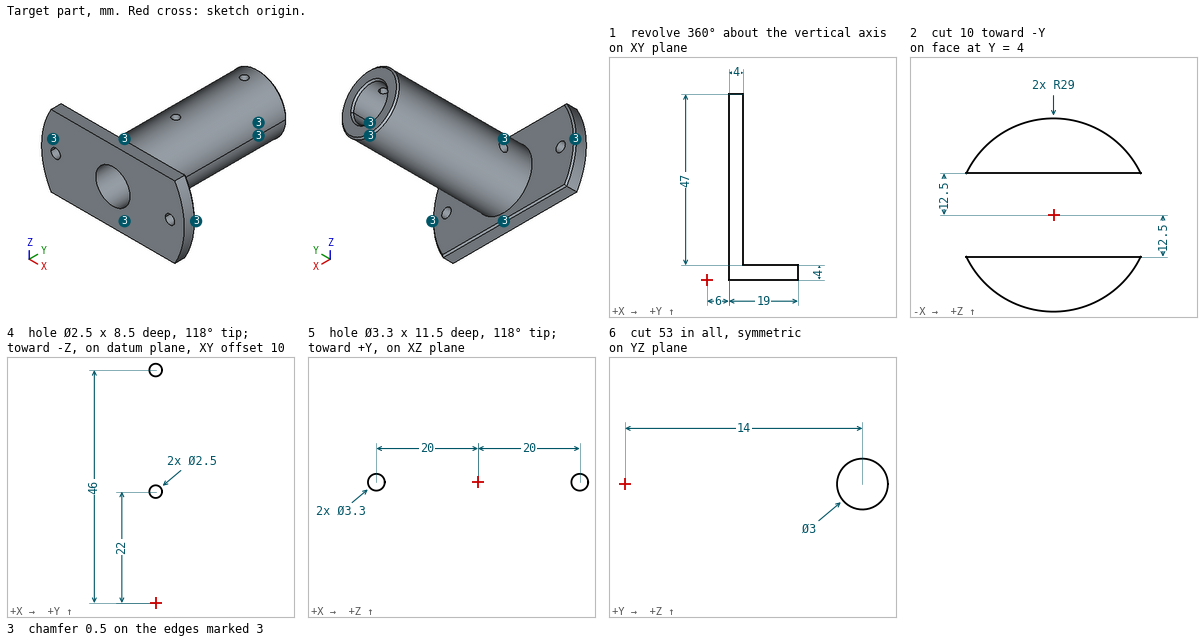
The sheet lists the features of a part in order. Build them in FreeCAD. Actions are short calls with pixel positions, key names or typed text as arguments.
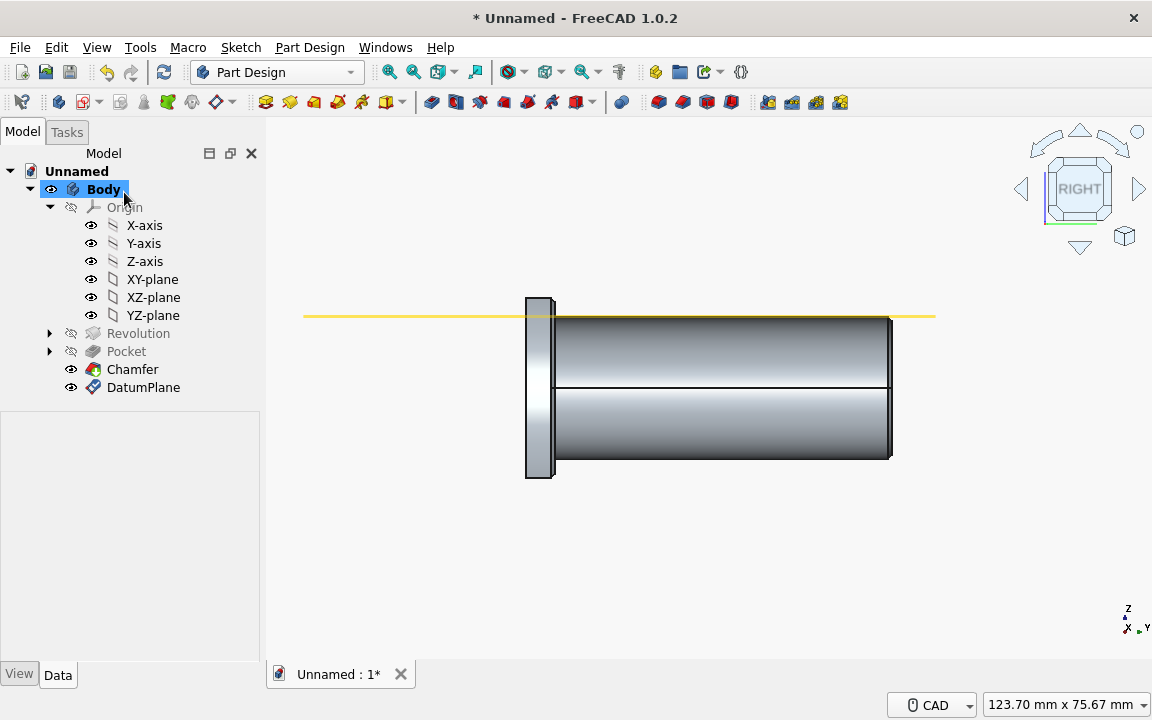
click(116, 387)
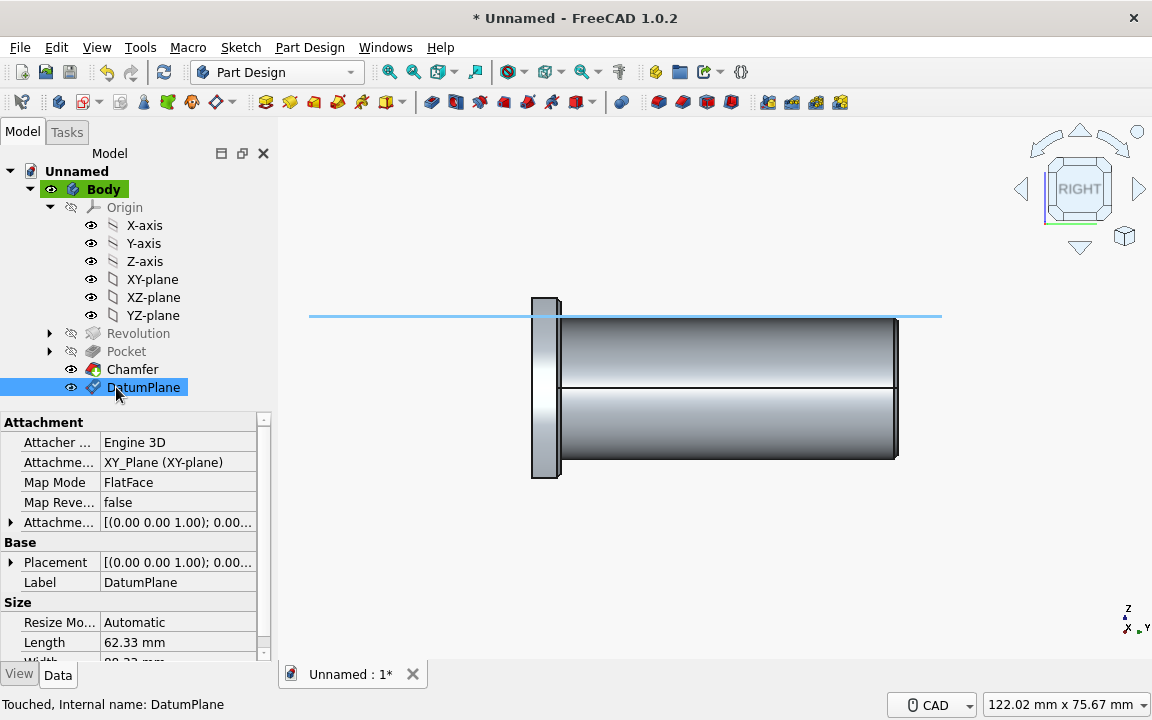
click(84, 102)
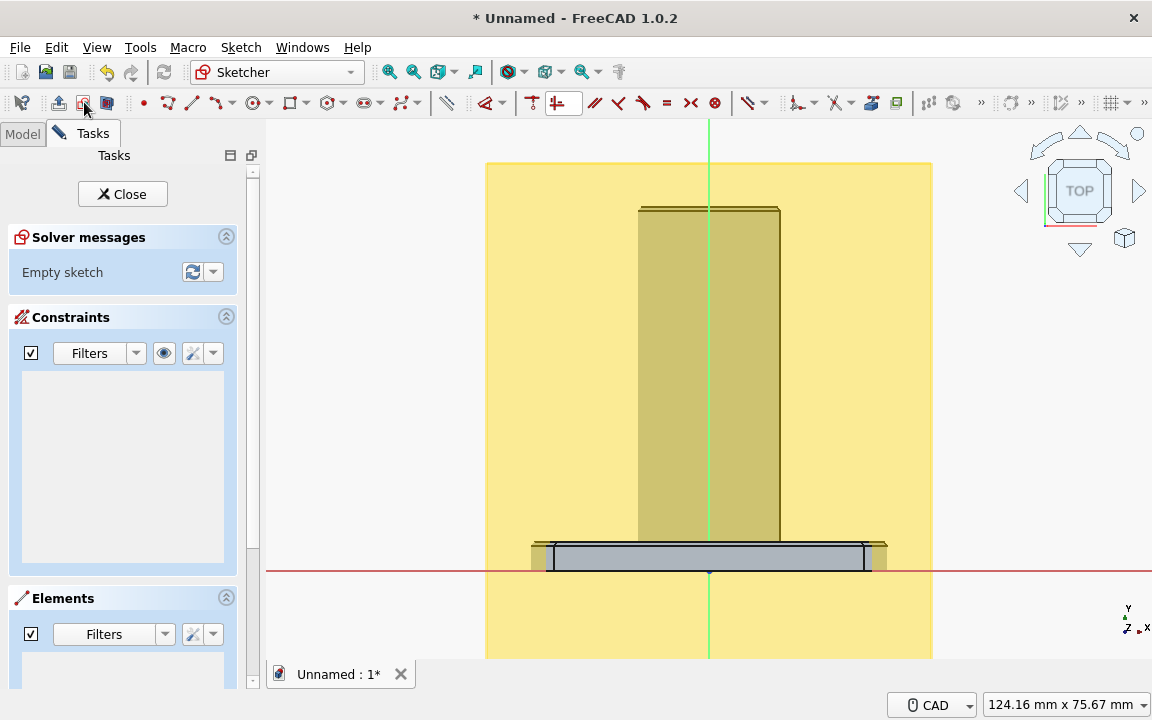
key(q)
key(s)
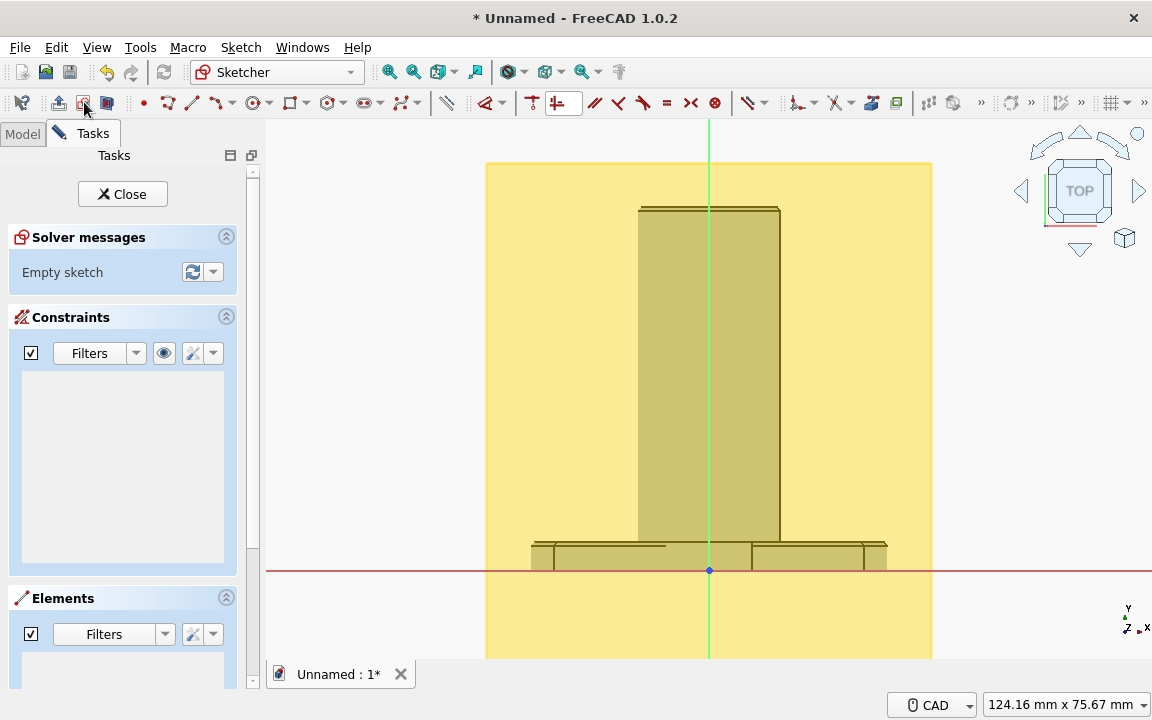
click(254, 104)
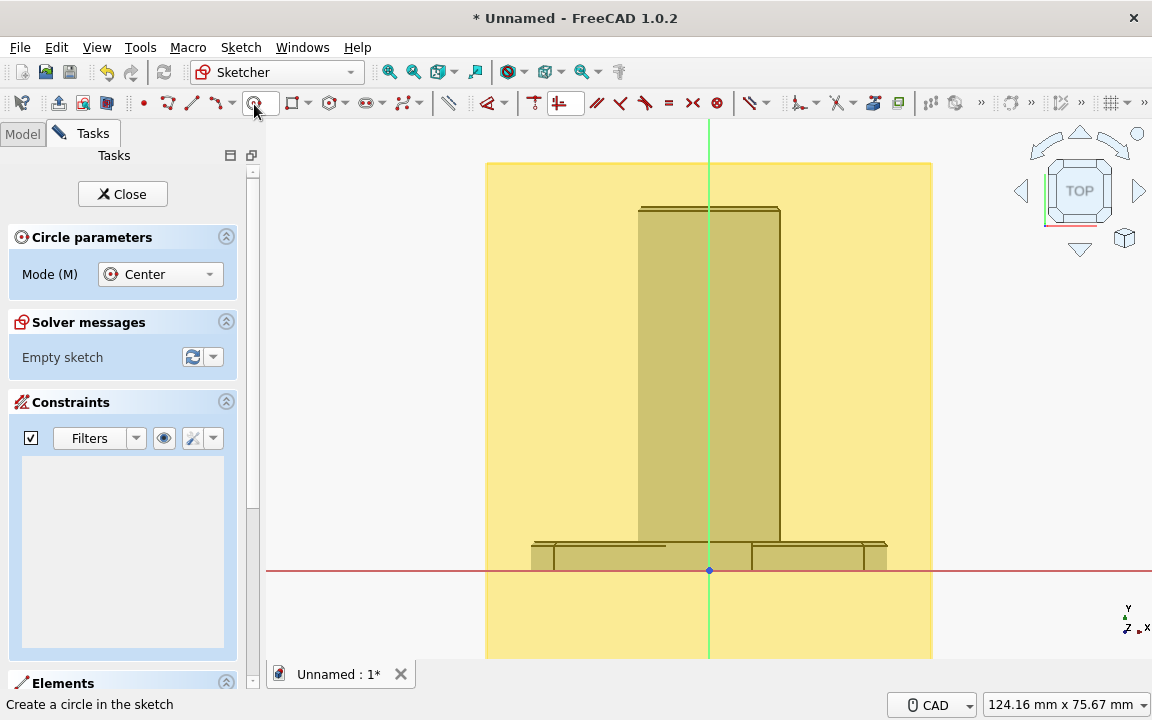
scroll(709, 414, up, 5)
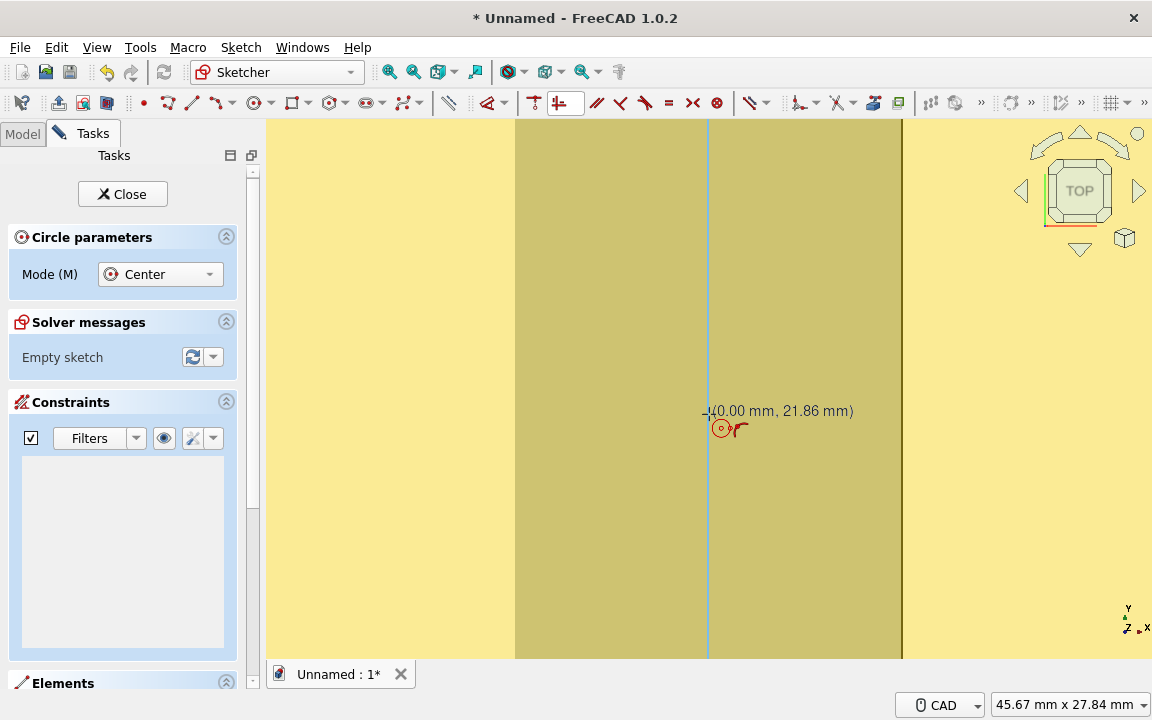
click(708, 413)
move(725, 396)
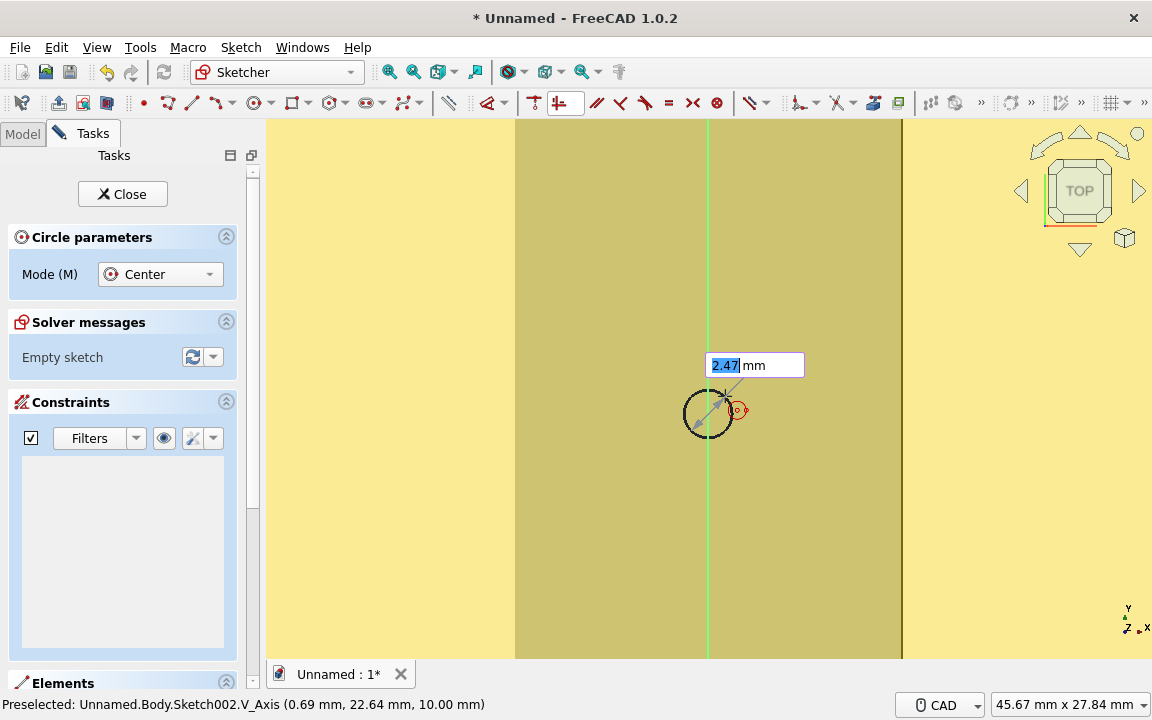
text(2.5)
key(Return)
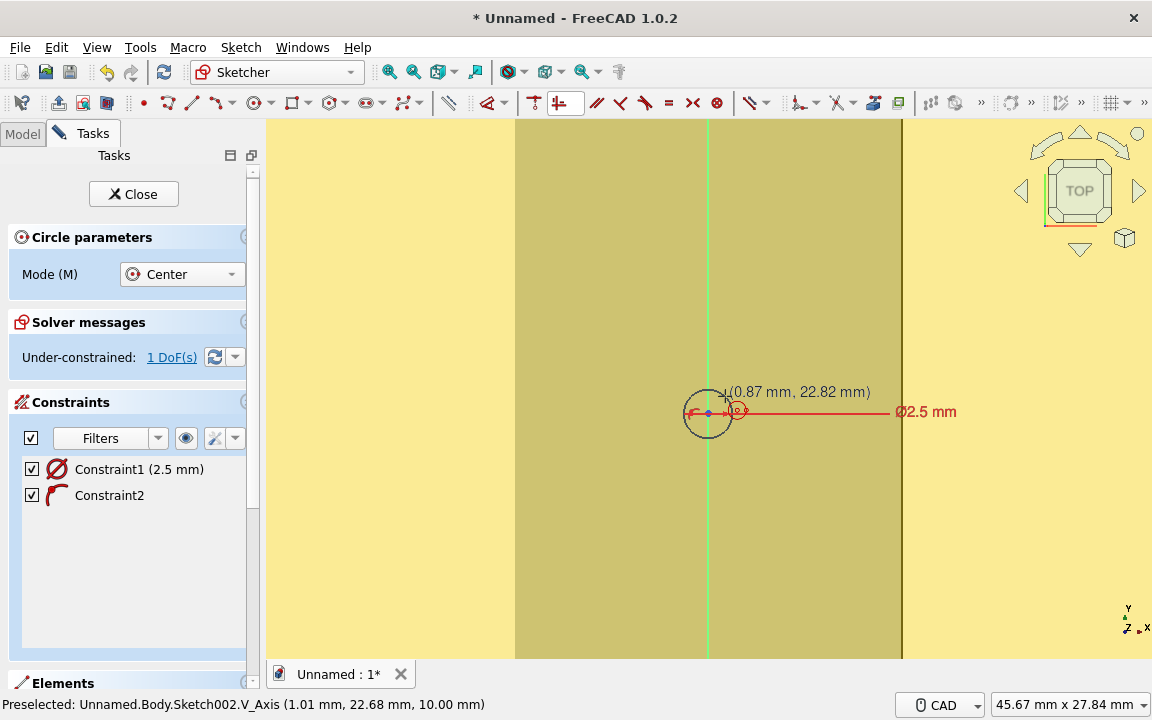
scroll(601, 393, down, 5)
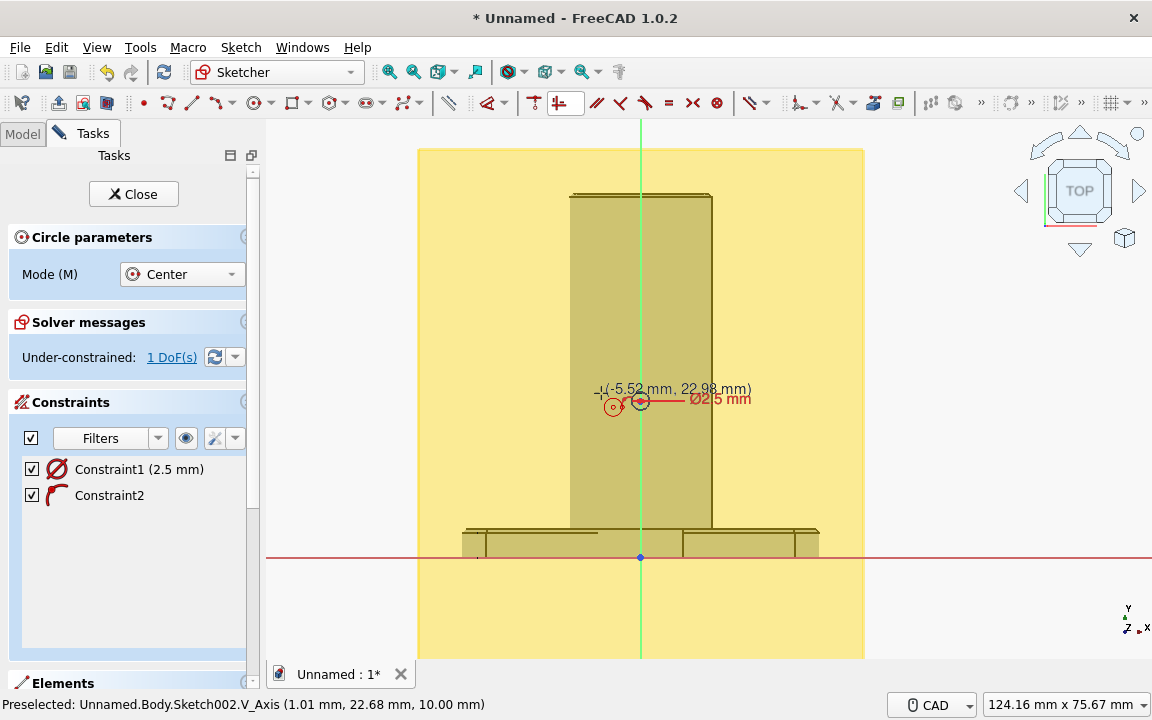
scroll(641, 229, up, 5)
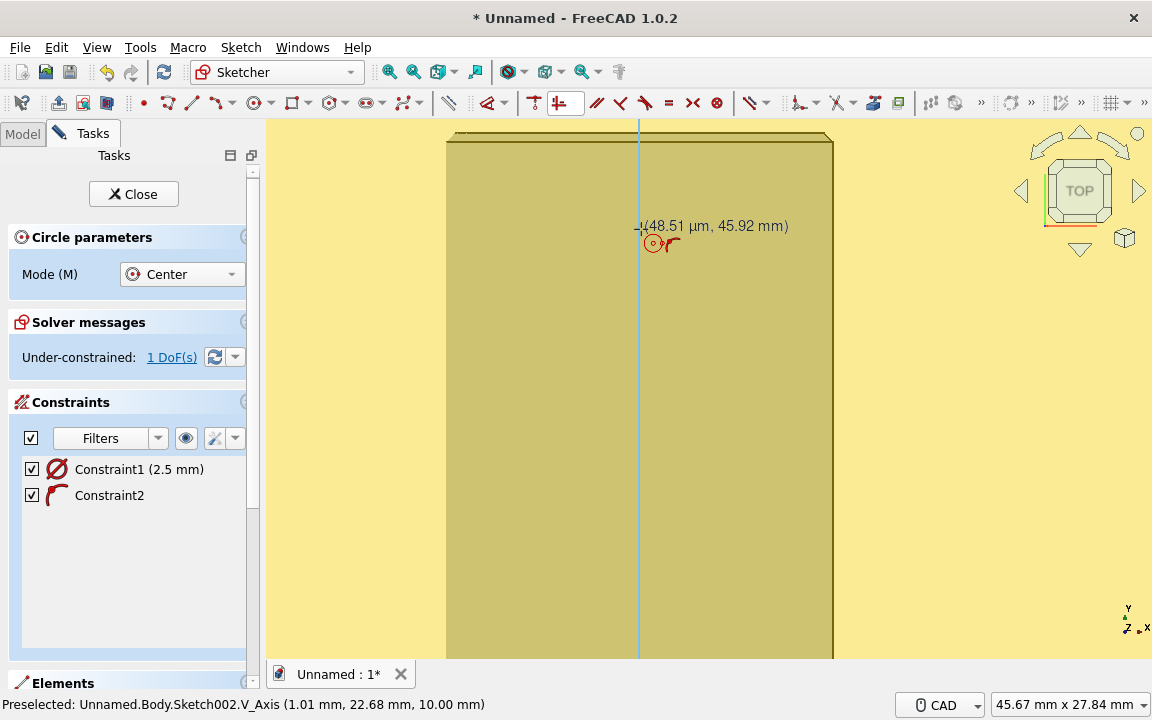
click(639, 230)
move(656, 213)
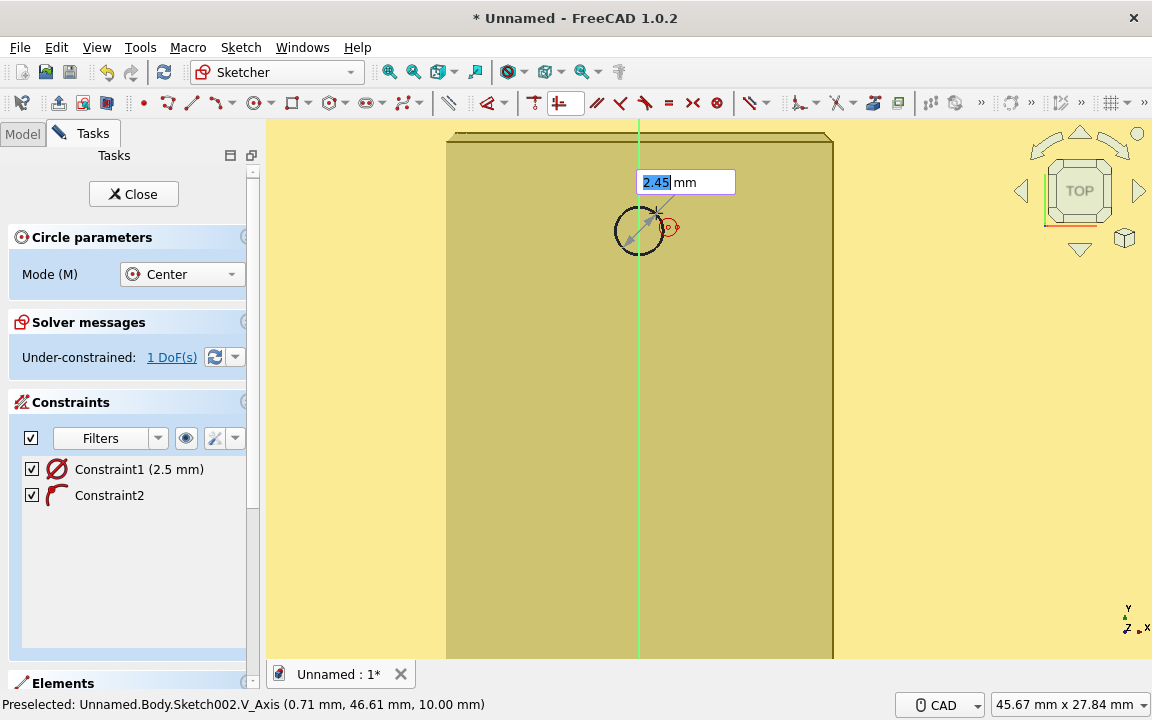
text(2.5)
key(Return)
key(Escape)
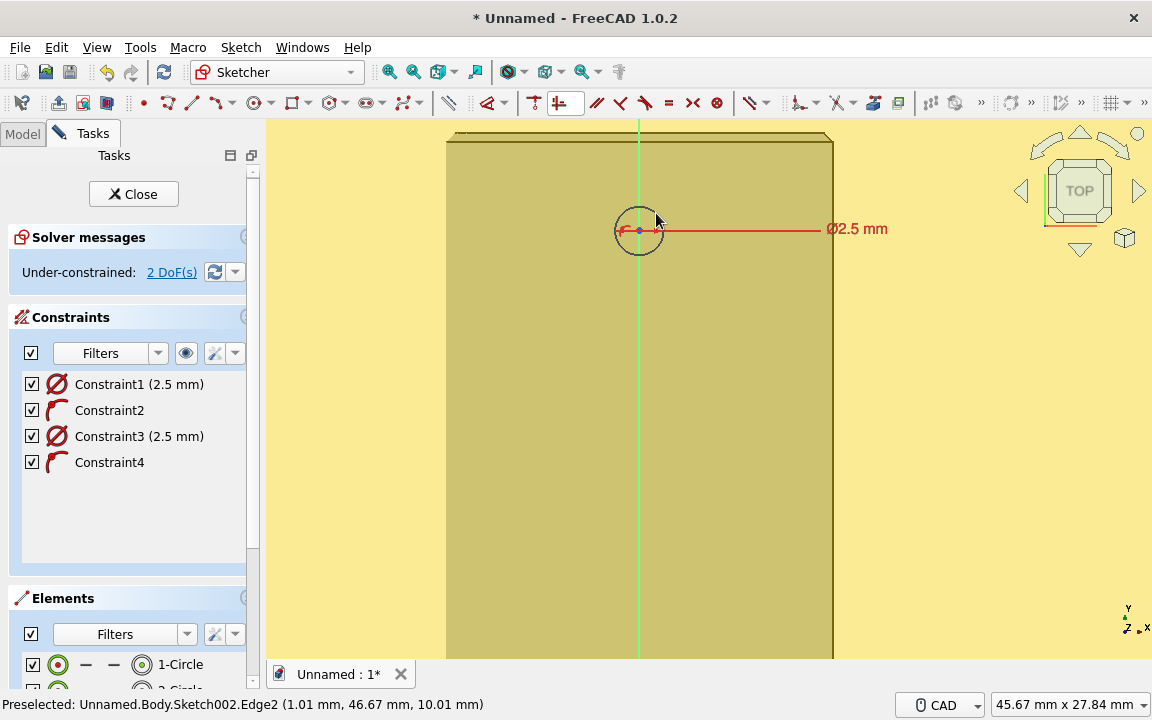
click(488, 104)